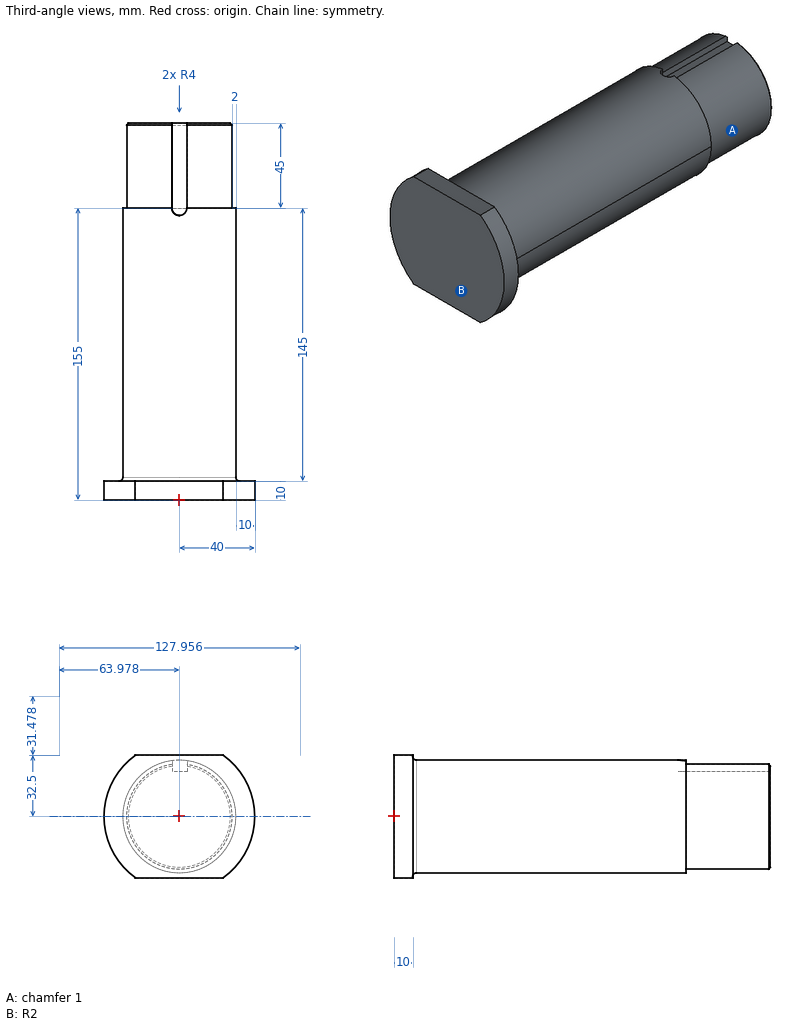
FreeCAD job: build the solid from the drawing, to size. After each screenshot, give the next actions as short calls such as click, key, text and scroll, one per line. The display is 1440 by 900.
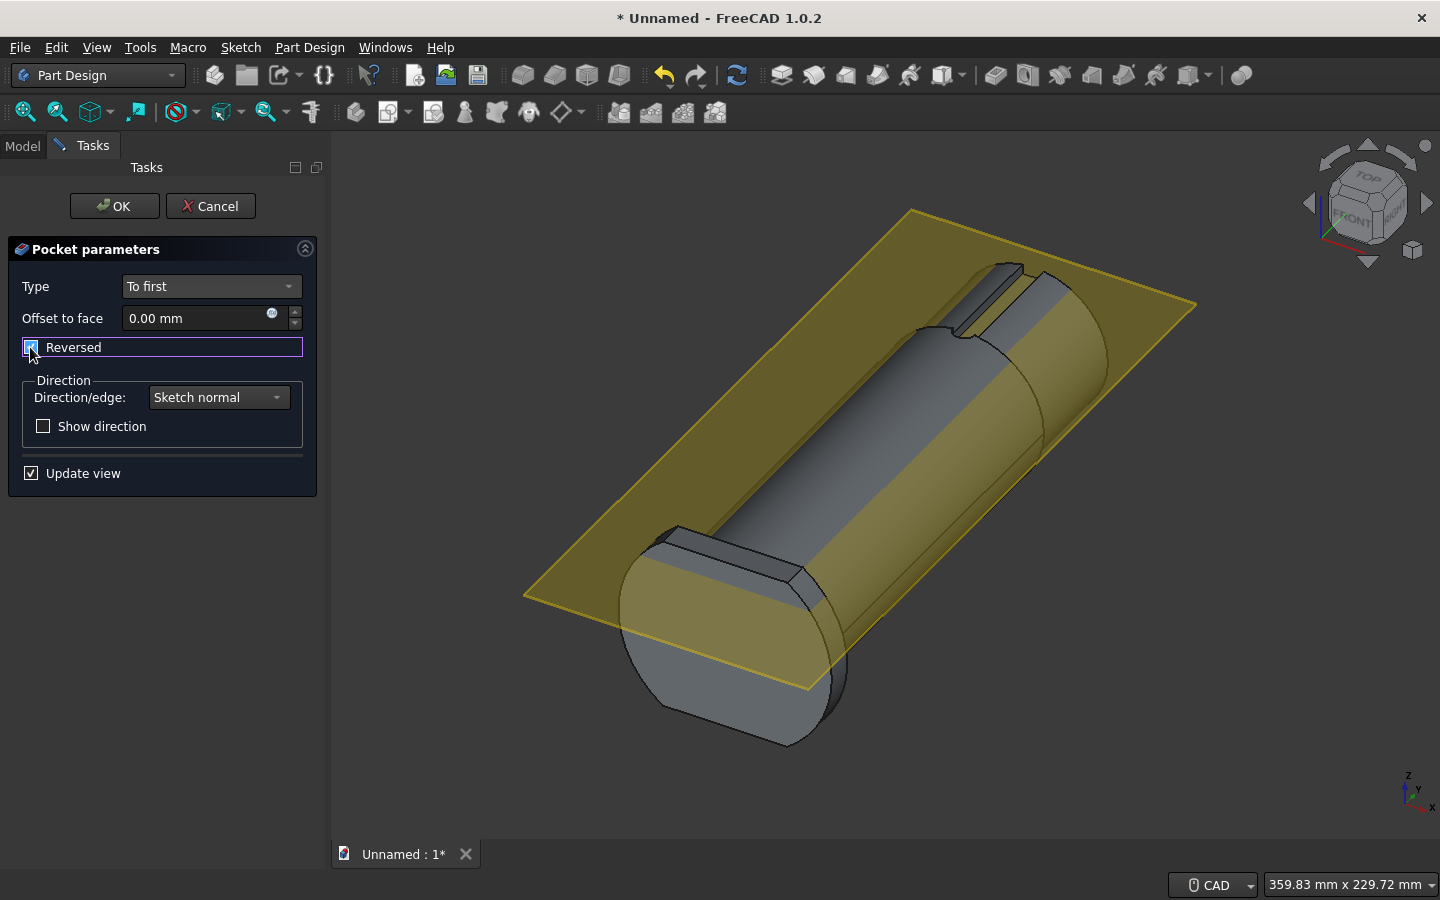
click(115, 206)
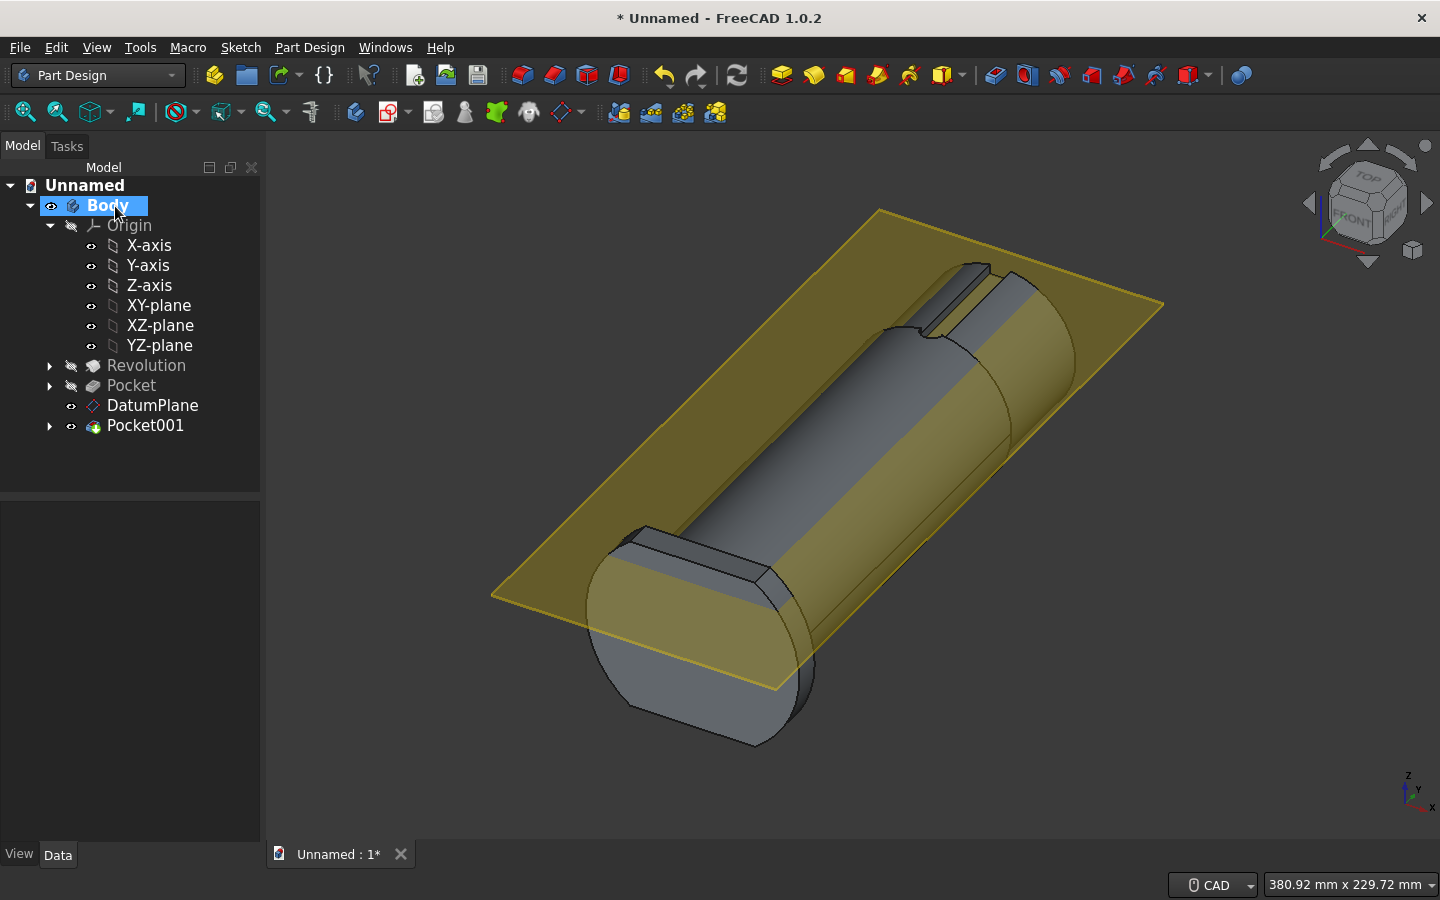
click(116, 406)
key(space)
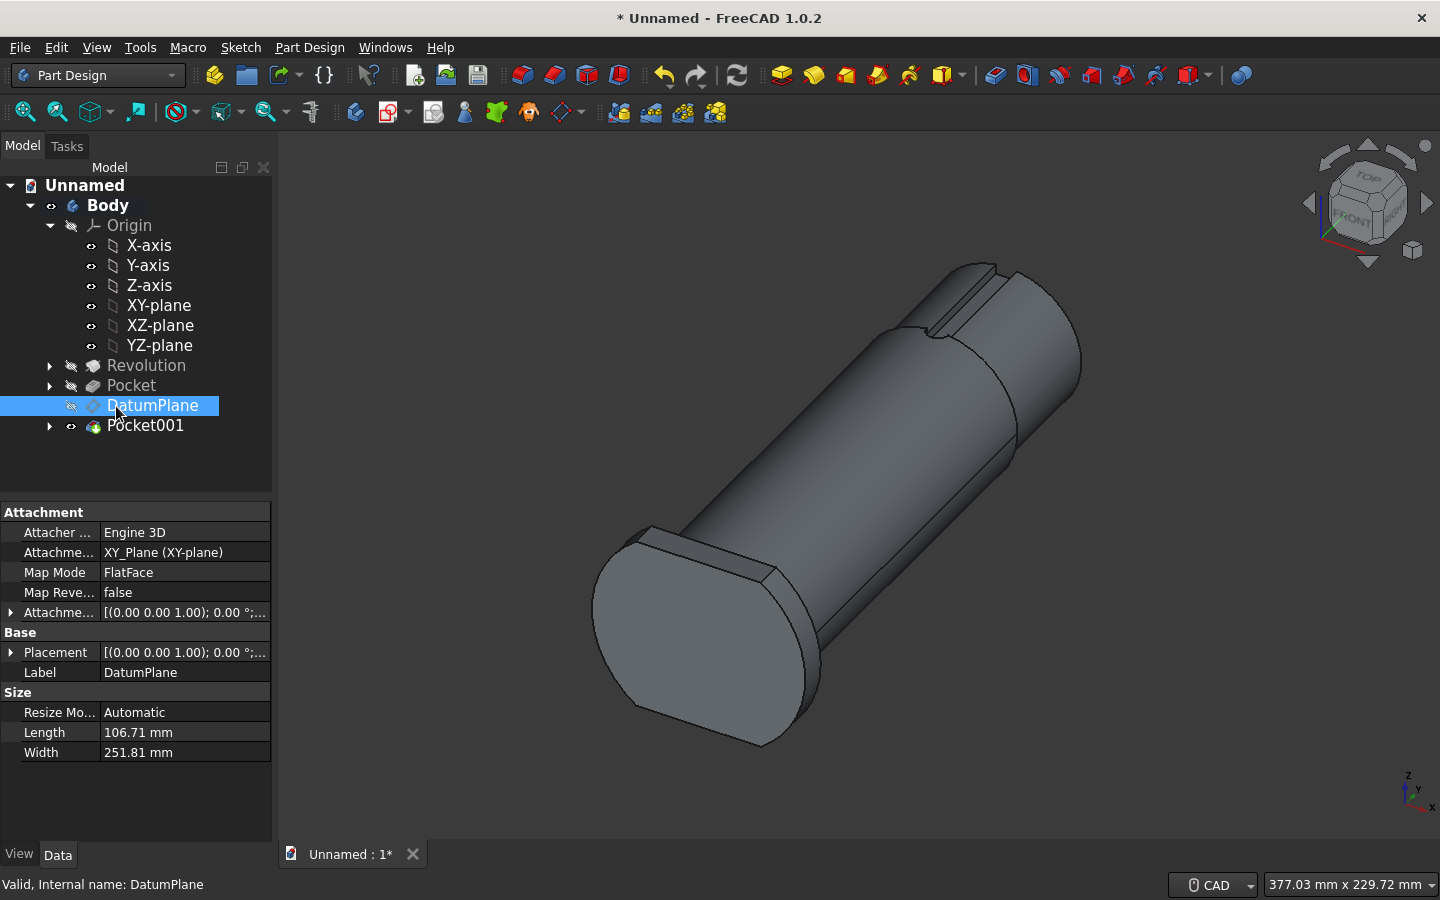
key(0)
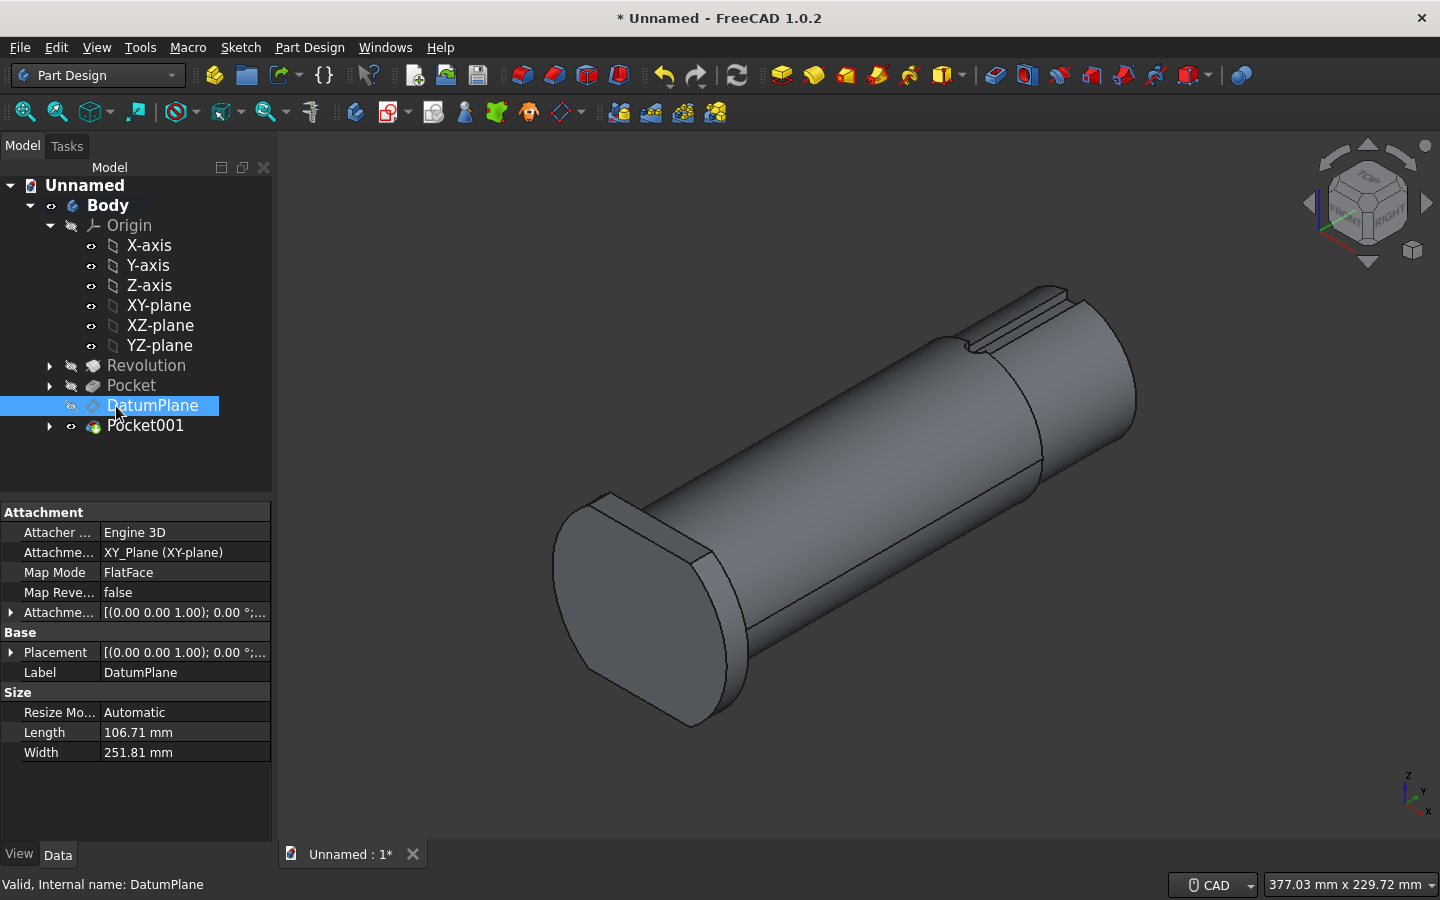
key(2)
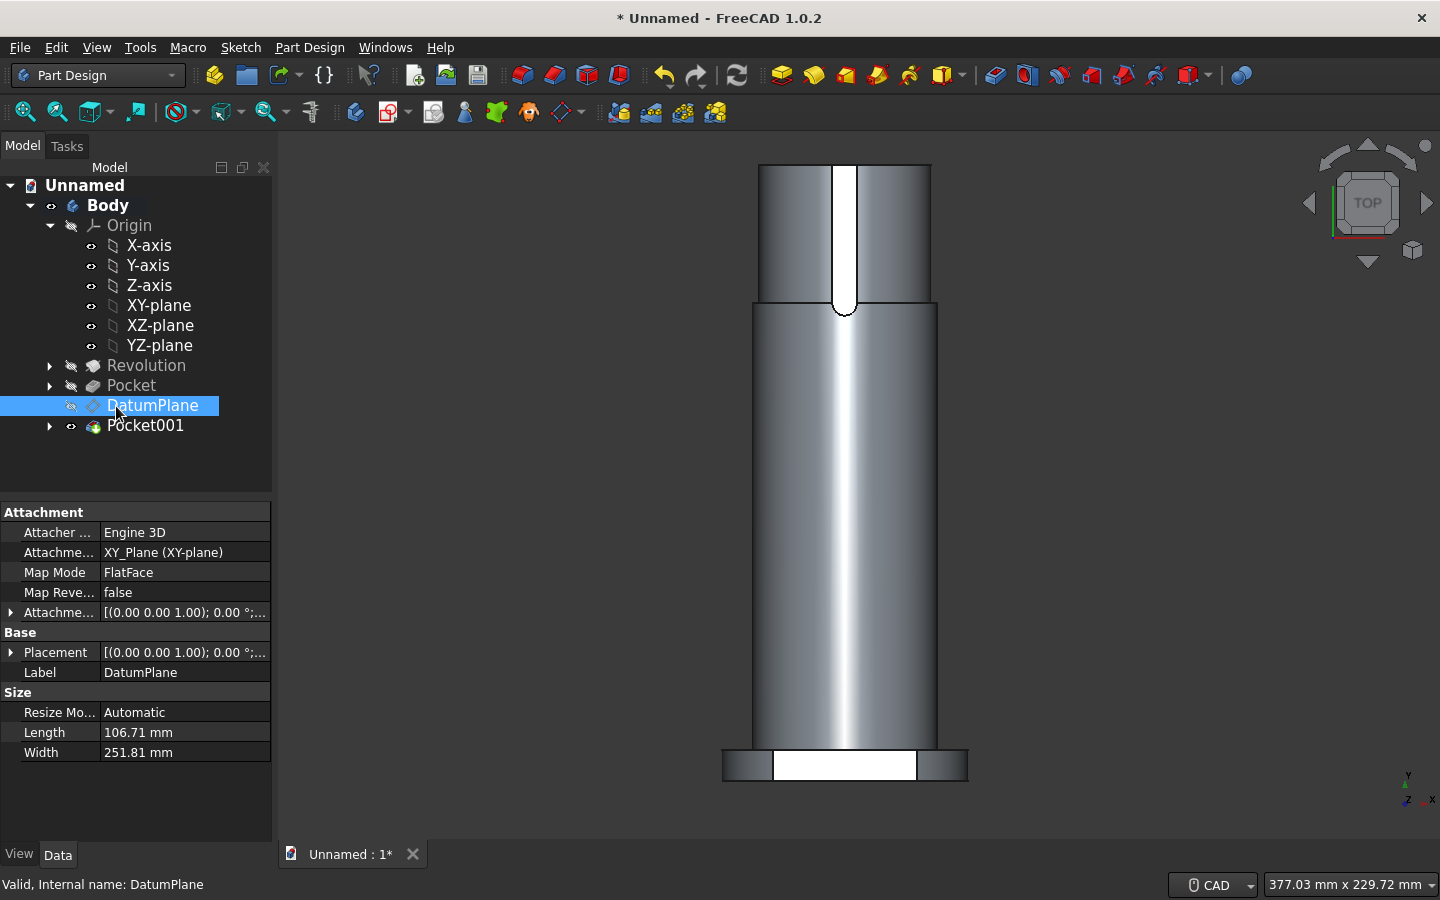
click(788, 164)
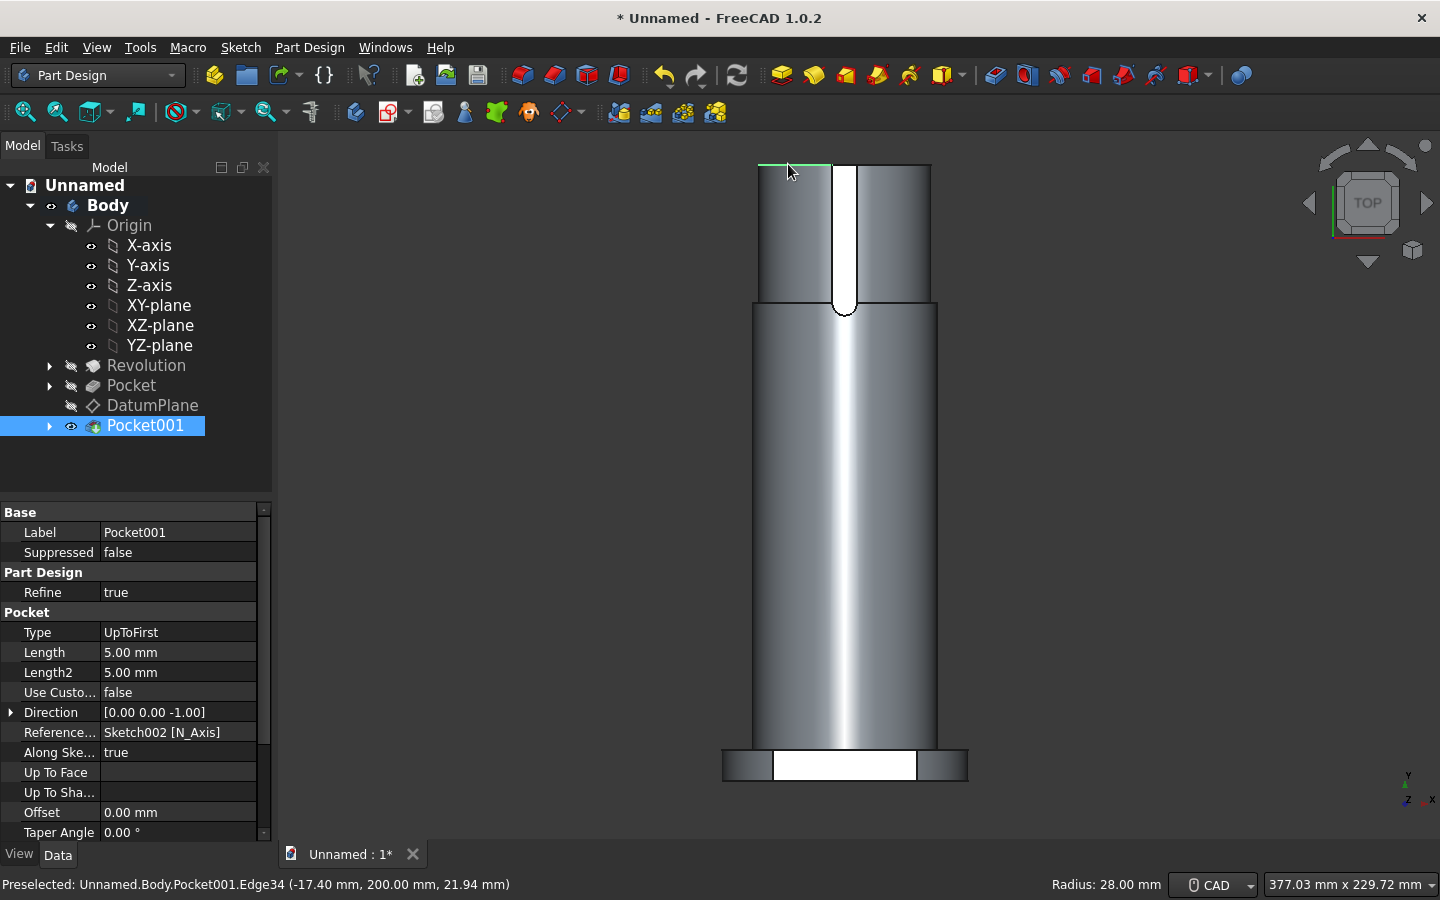
click(556, 76)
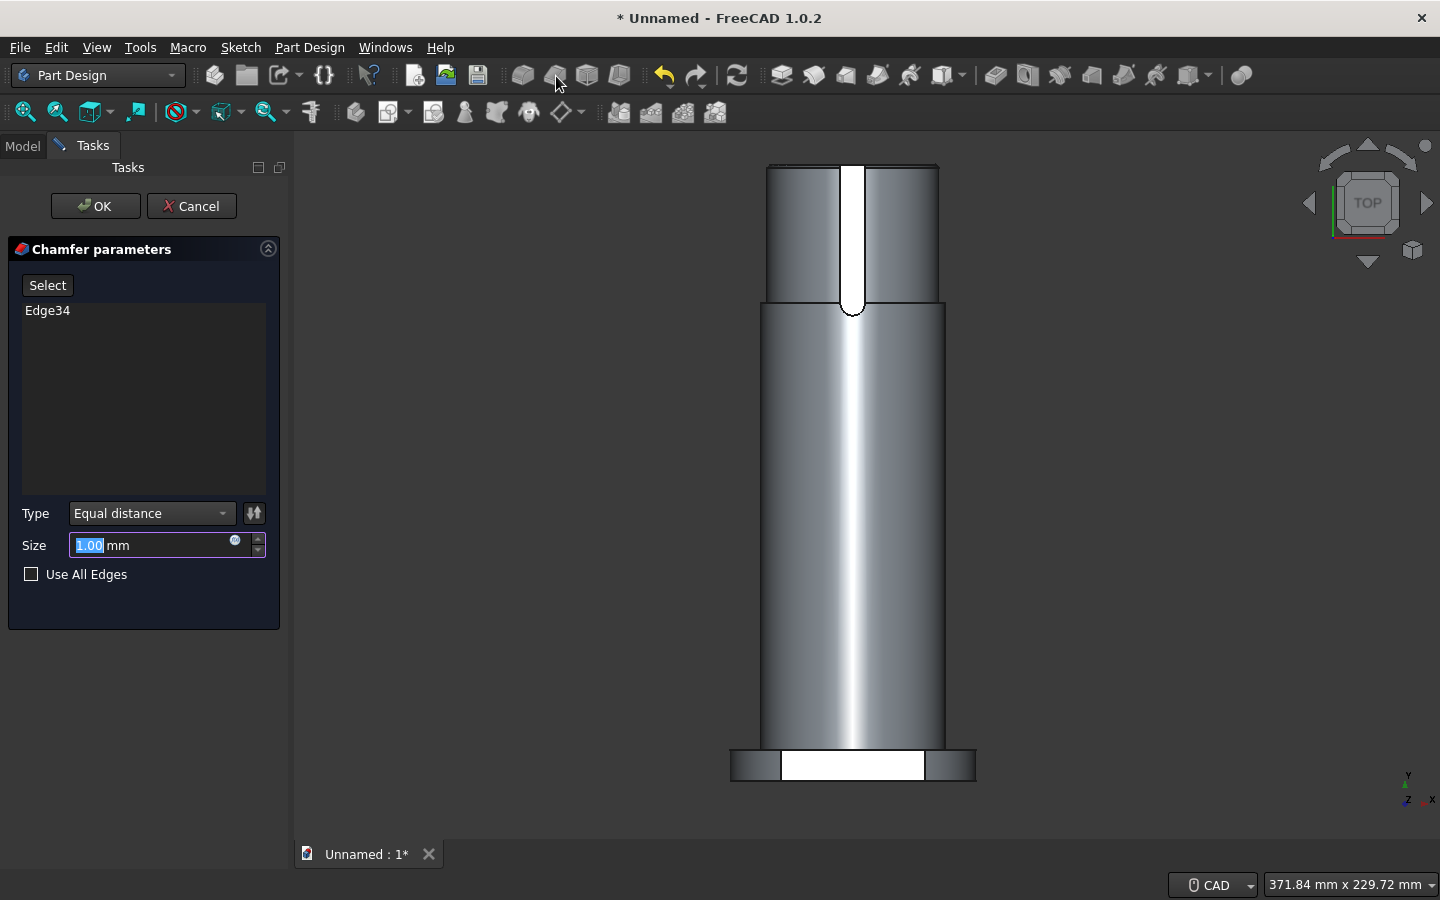
text(1)
key(Tab)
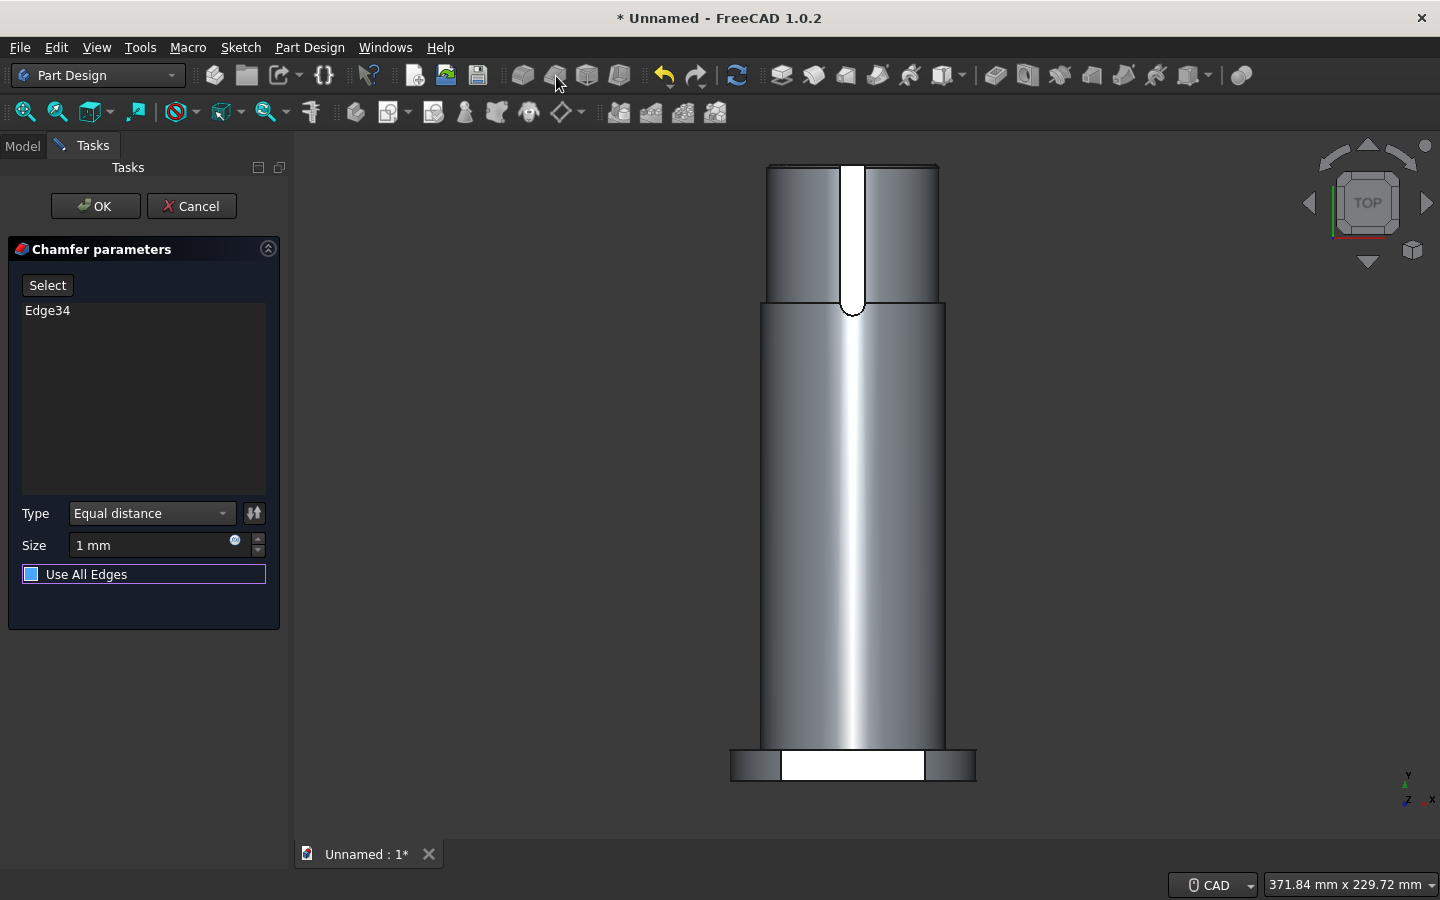
click(96, 206)